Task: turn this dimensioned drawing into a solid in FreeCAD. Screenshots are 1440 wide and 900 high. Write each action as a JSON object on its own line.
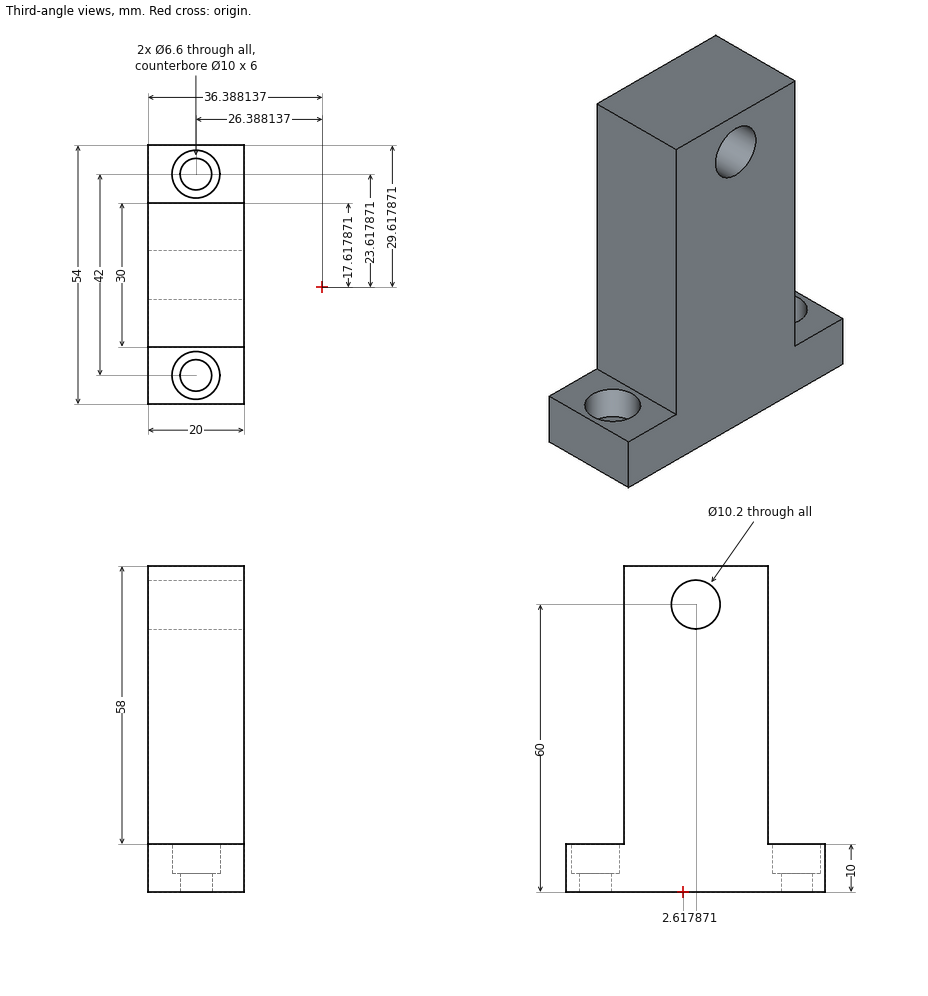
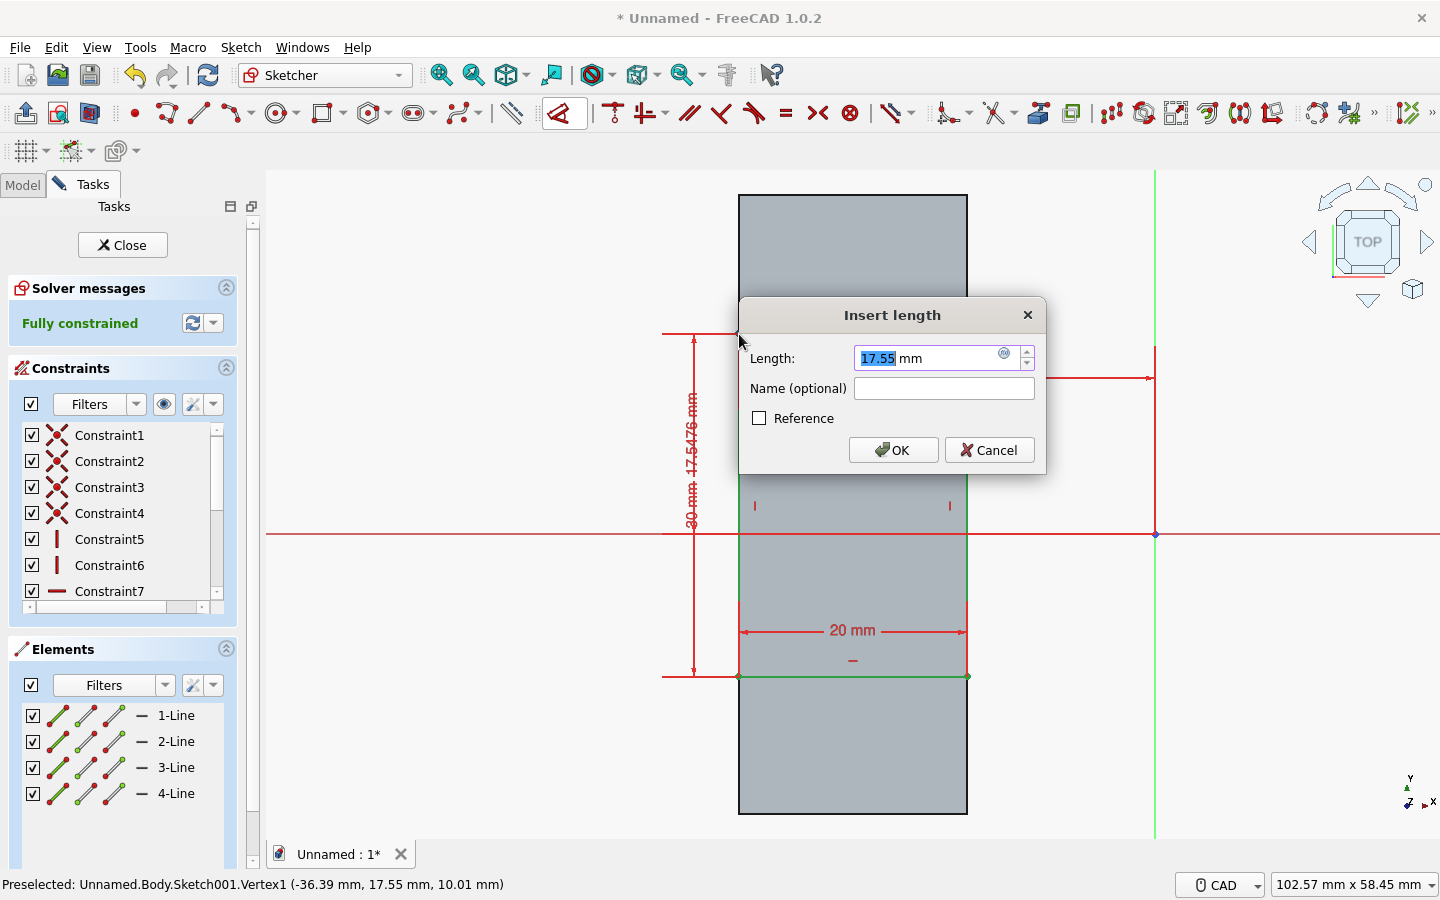
{"action": "type", "text": "17.617871"}
{"action": "key", "text": "Return"}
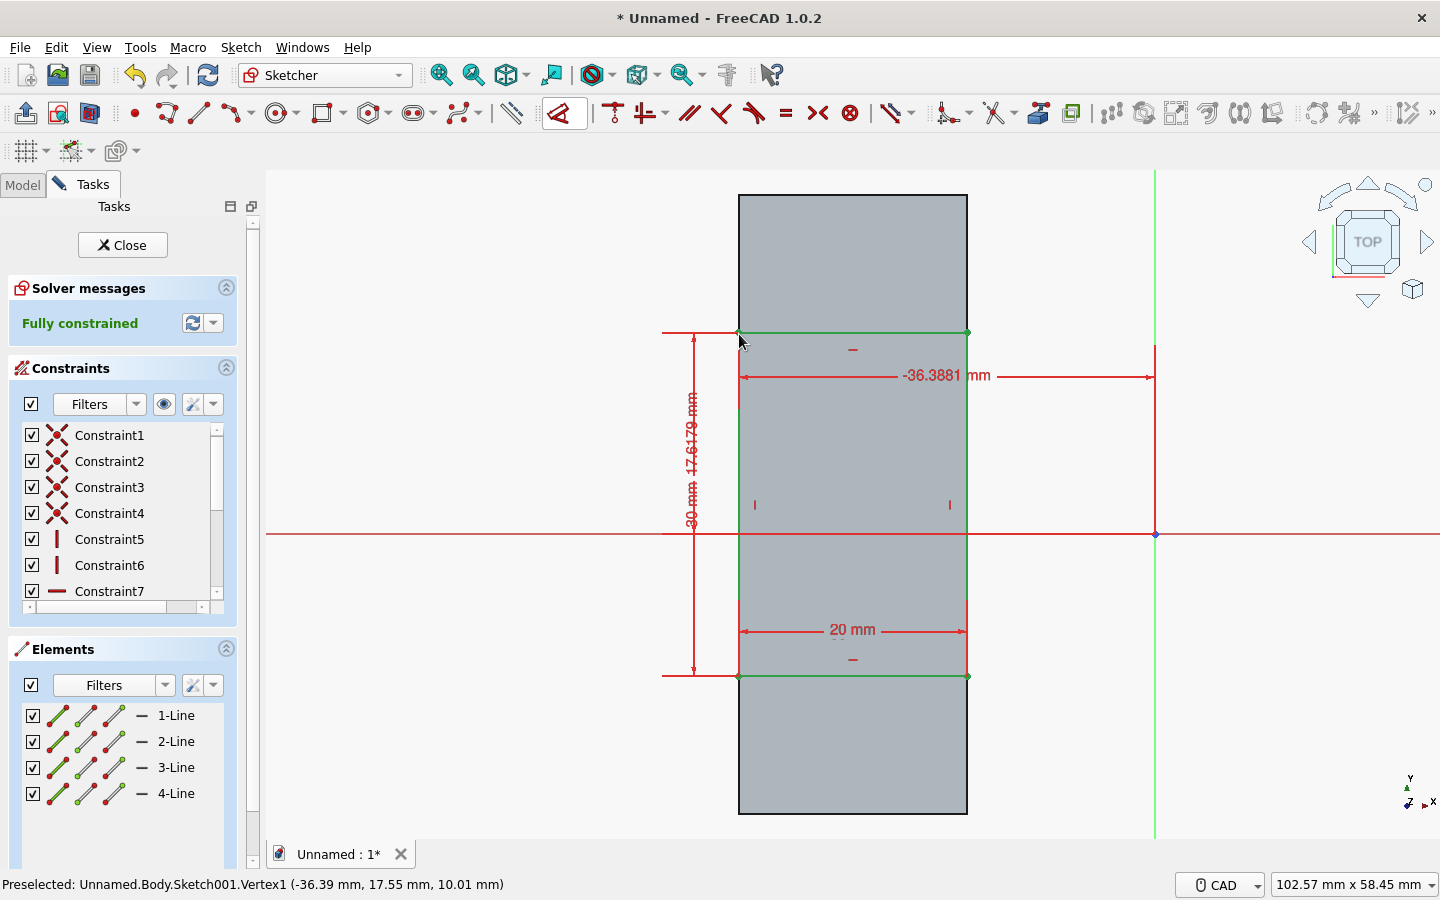
{"action": "left_click", "coordinate": [123, 245]}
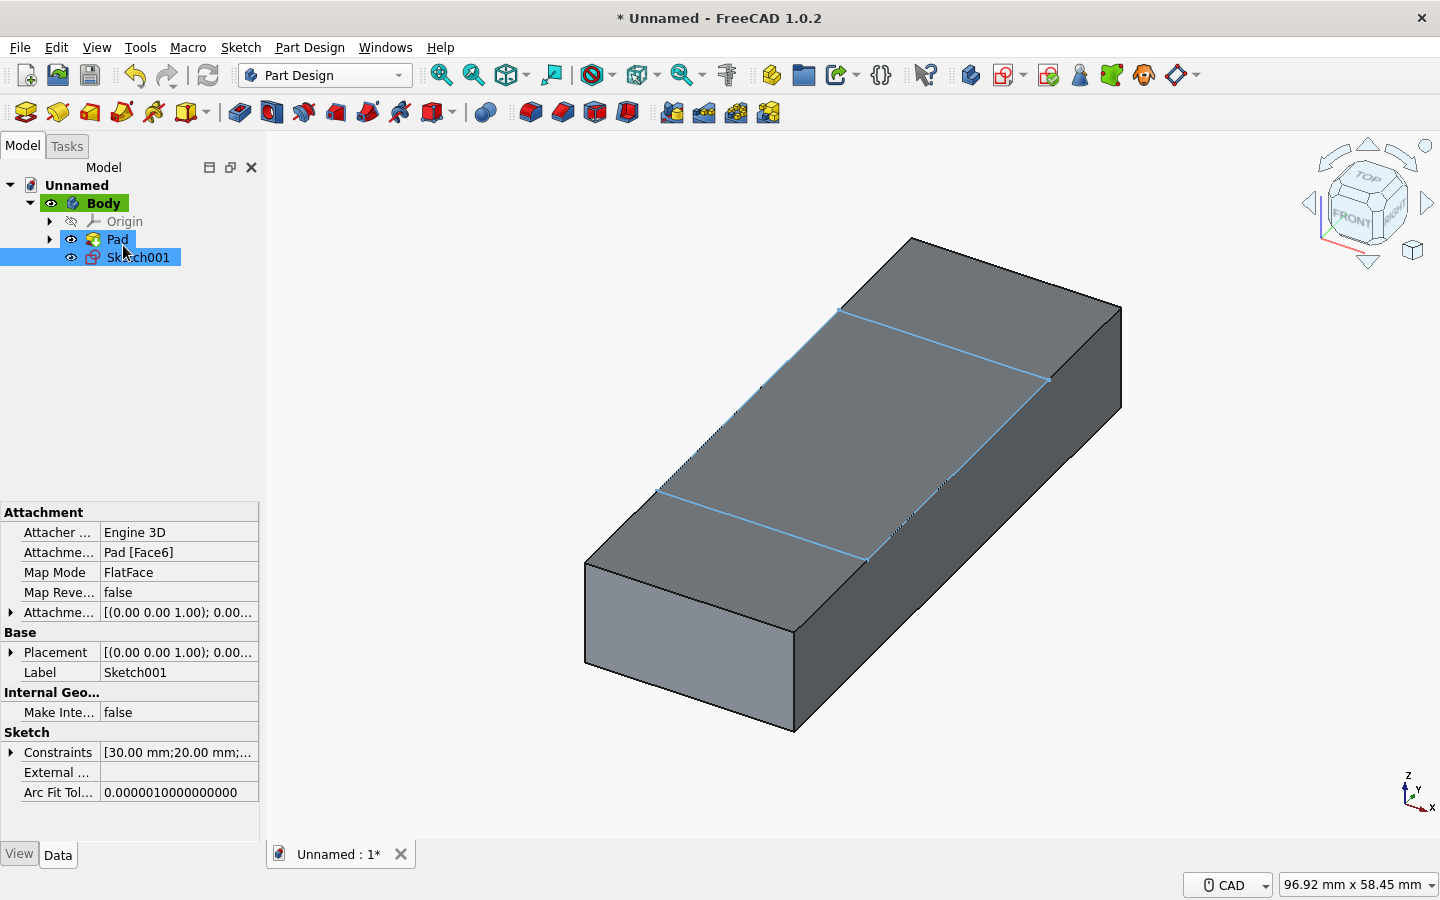
{"action": "left_click", "coordinate": [26, 112]}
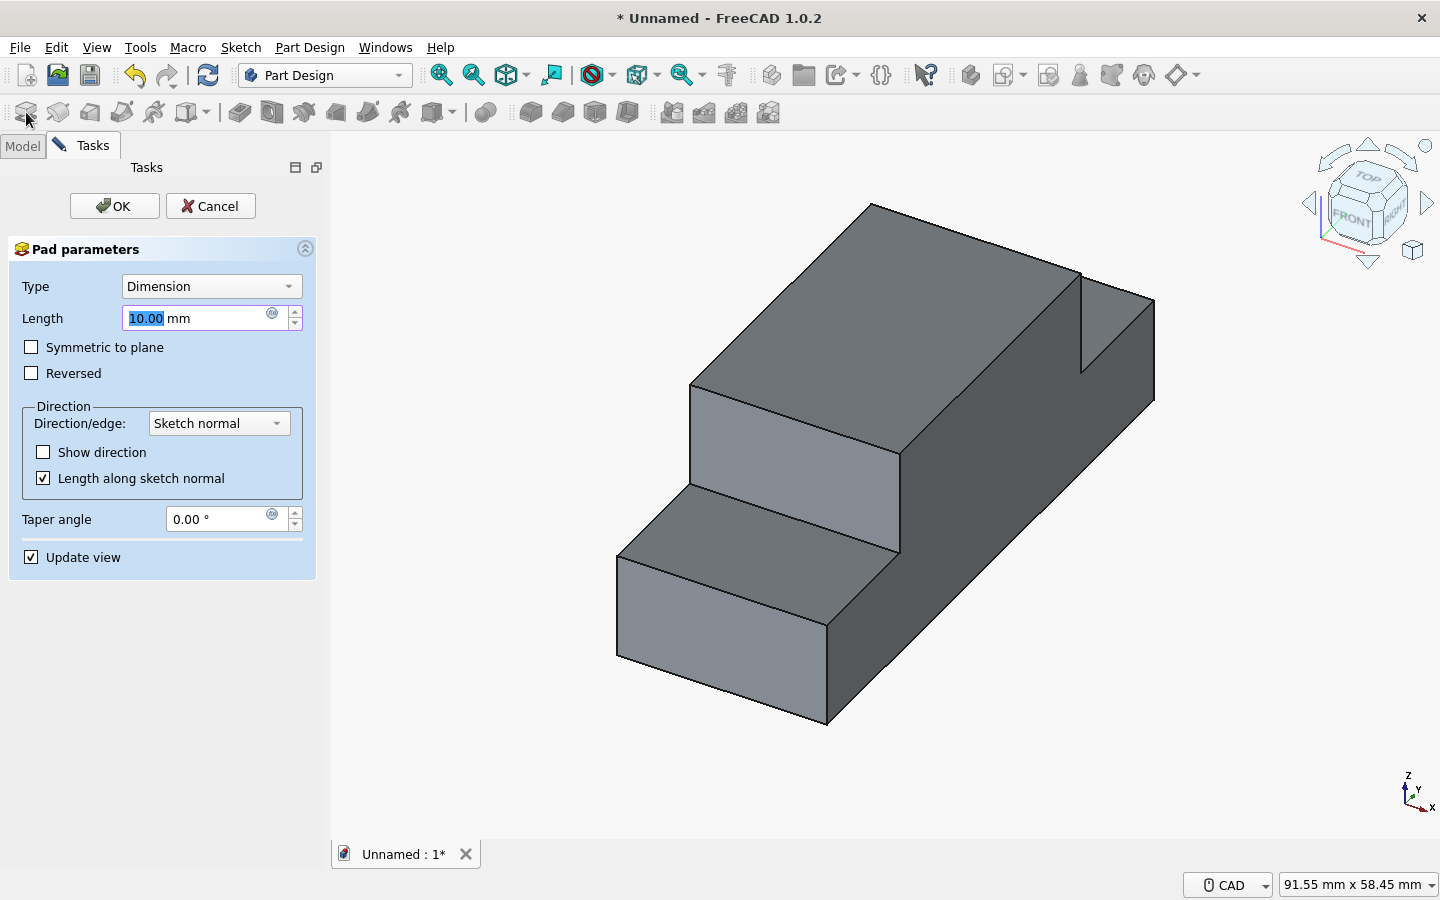
{"action": "type", "text": "58"}
{"action": "key", "text": "Tab"}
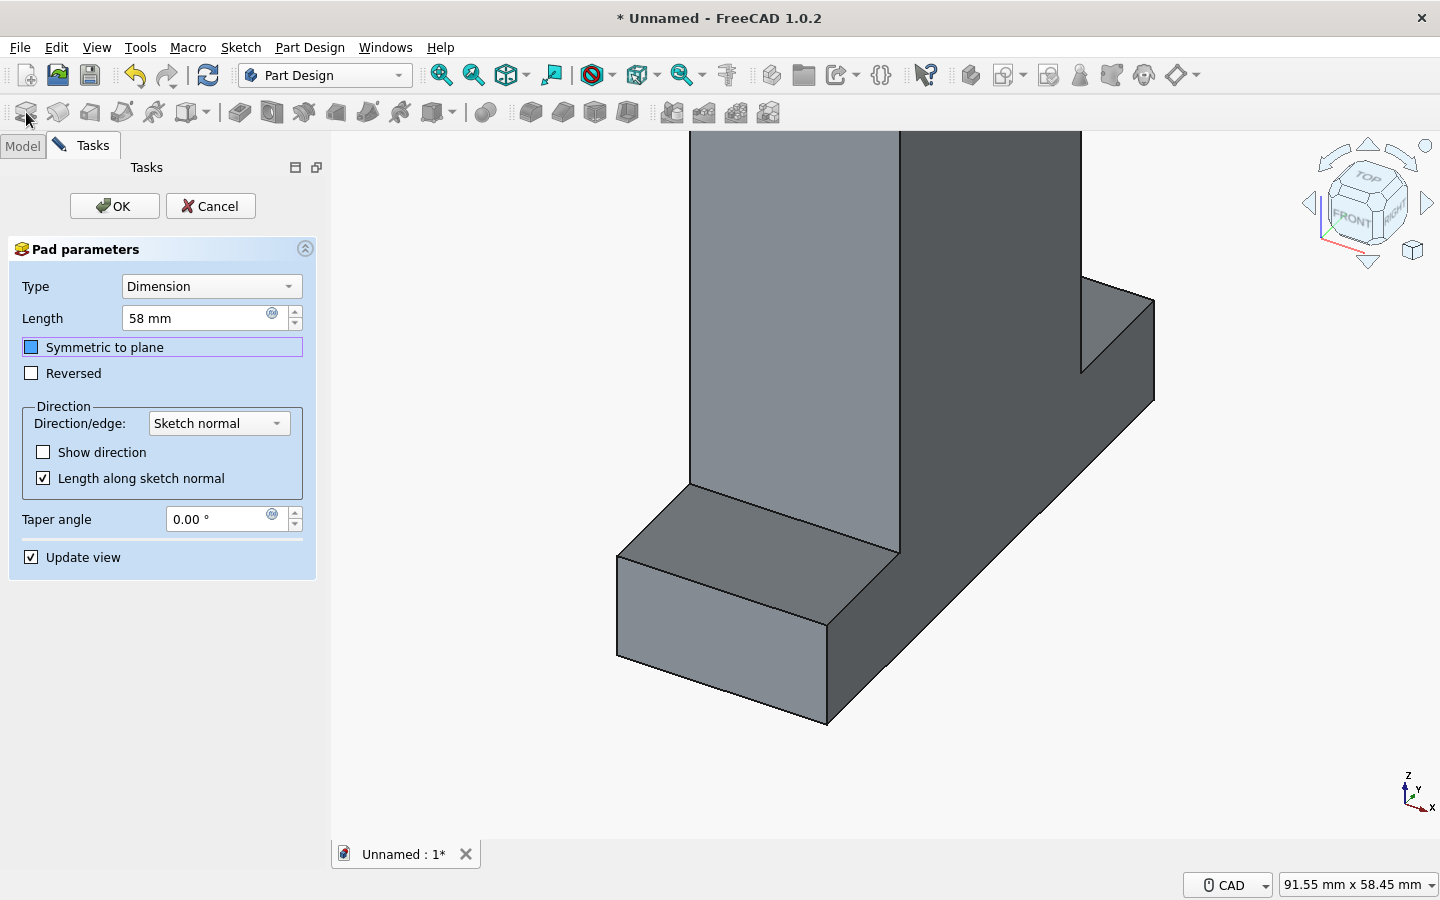
{"action": "left_click", "coordinate": [115, 206]}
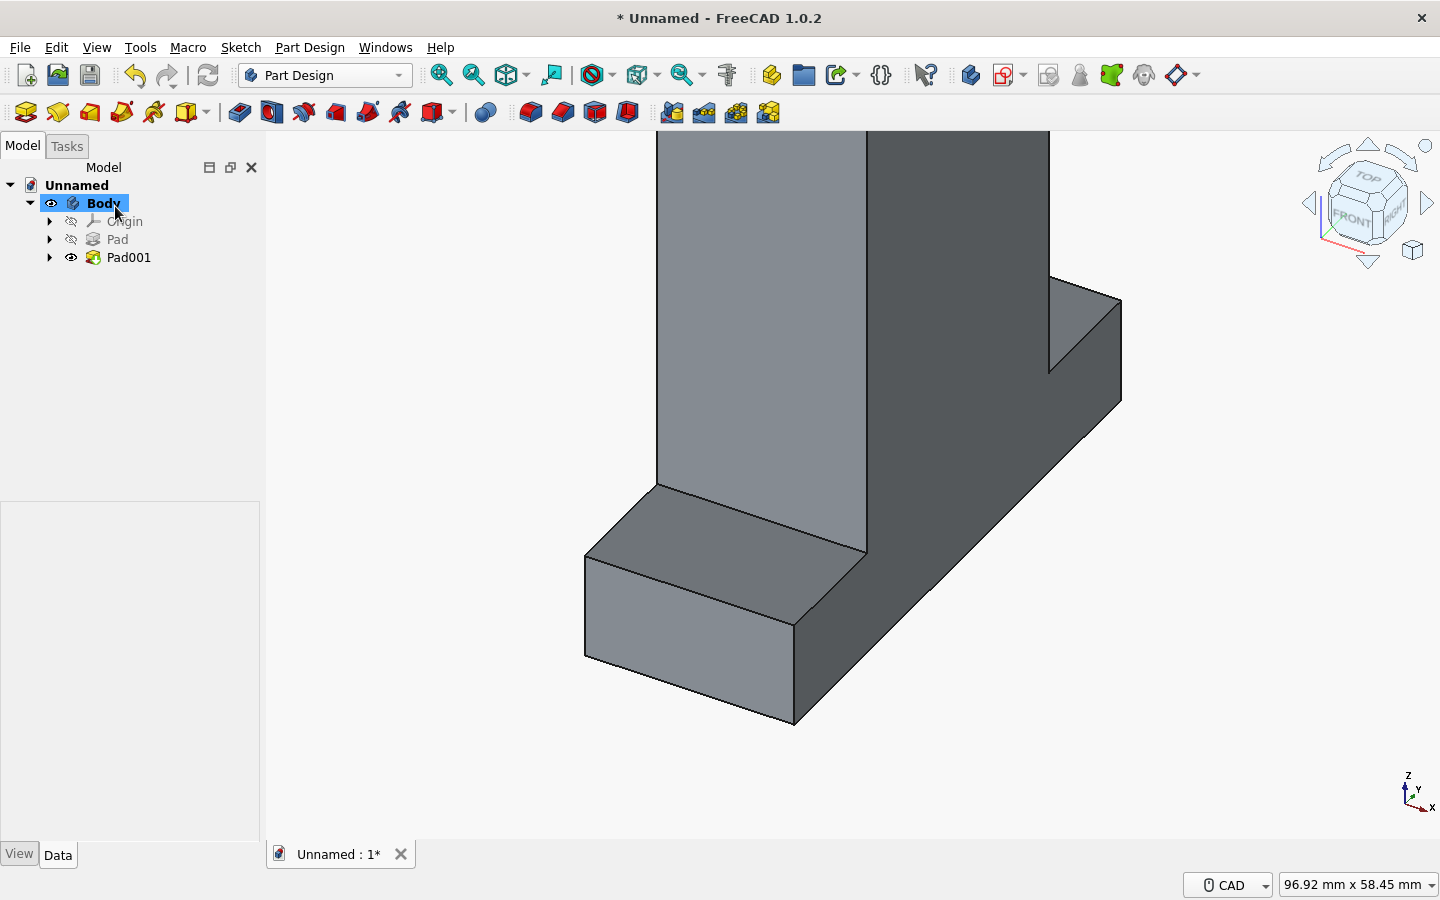
{"action": "left_click", "coordinate": [442, 76]}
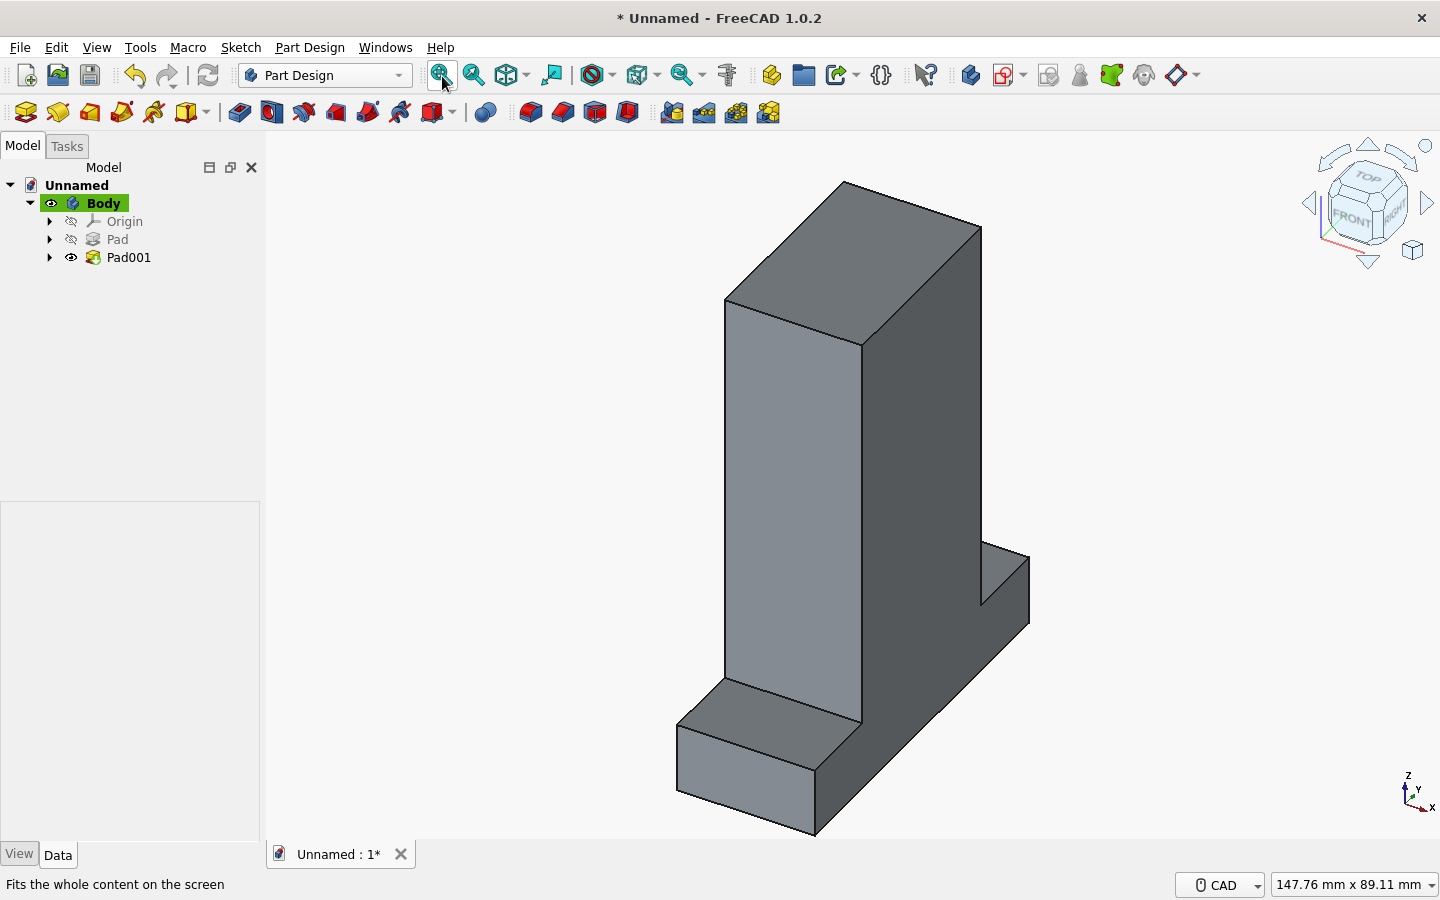
{"action": "left_click", "coordinate": [789, 730]}